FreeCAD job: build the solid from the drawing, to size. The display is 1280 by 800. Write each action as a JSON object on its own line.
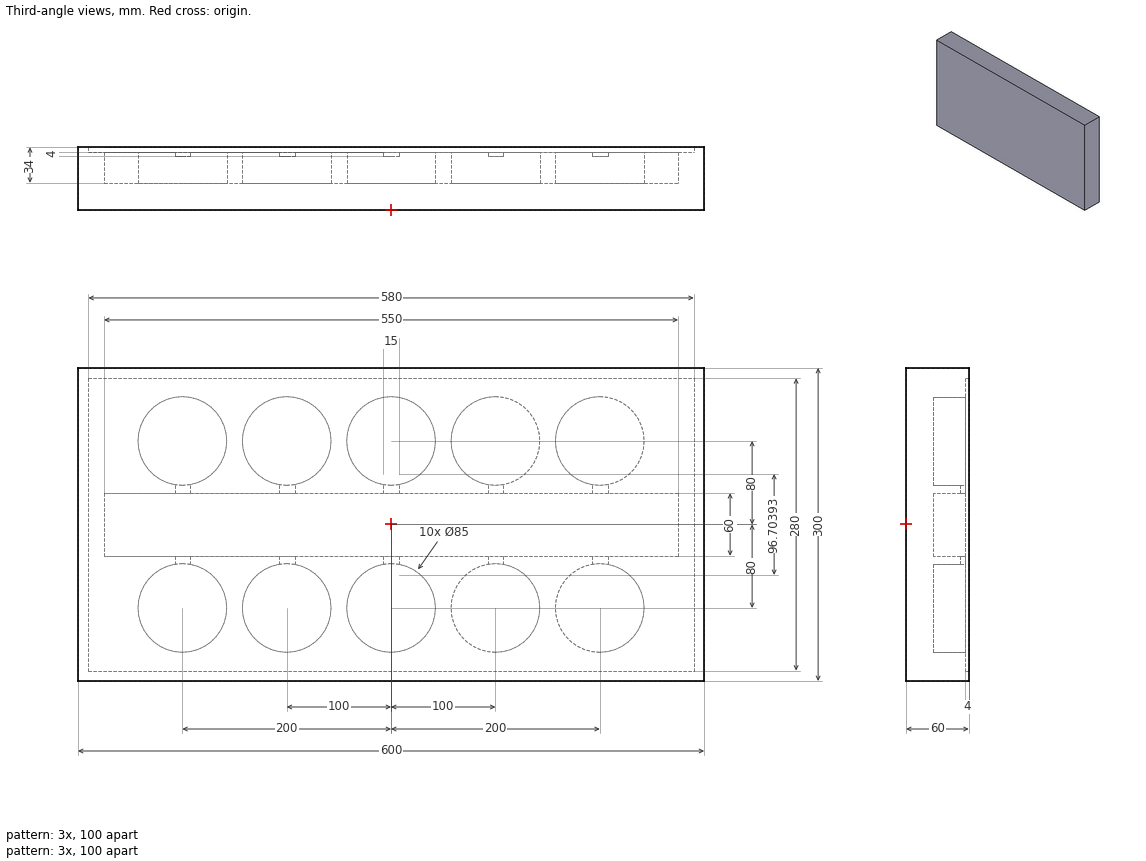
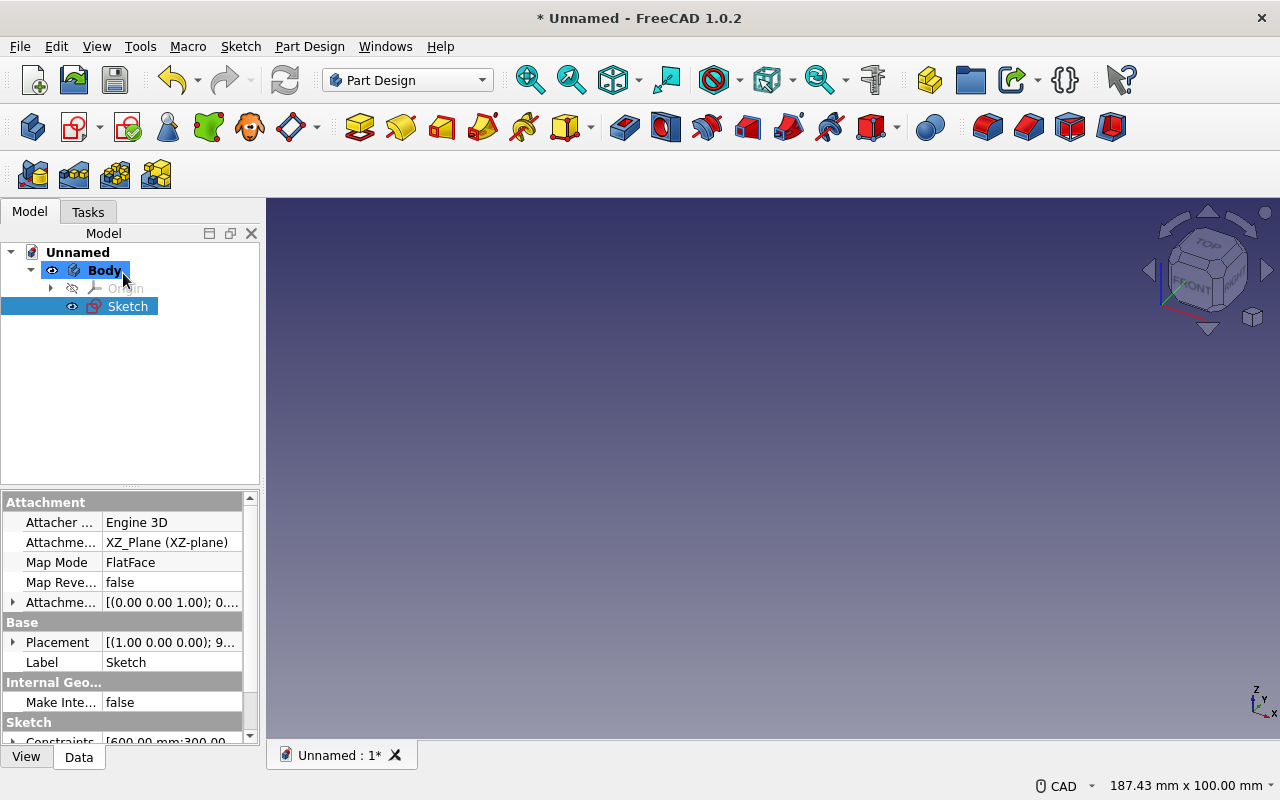
{"action": "left_click", "coordinate": [360, 128]}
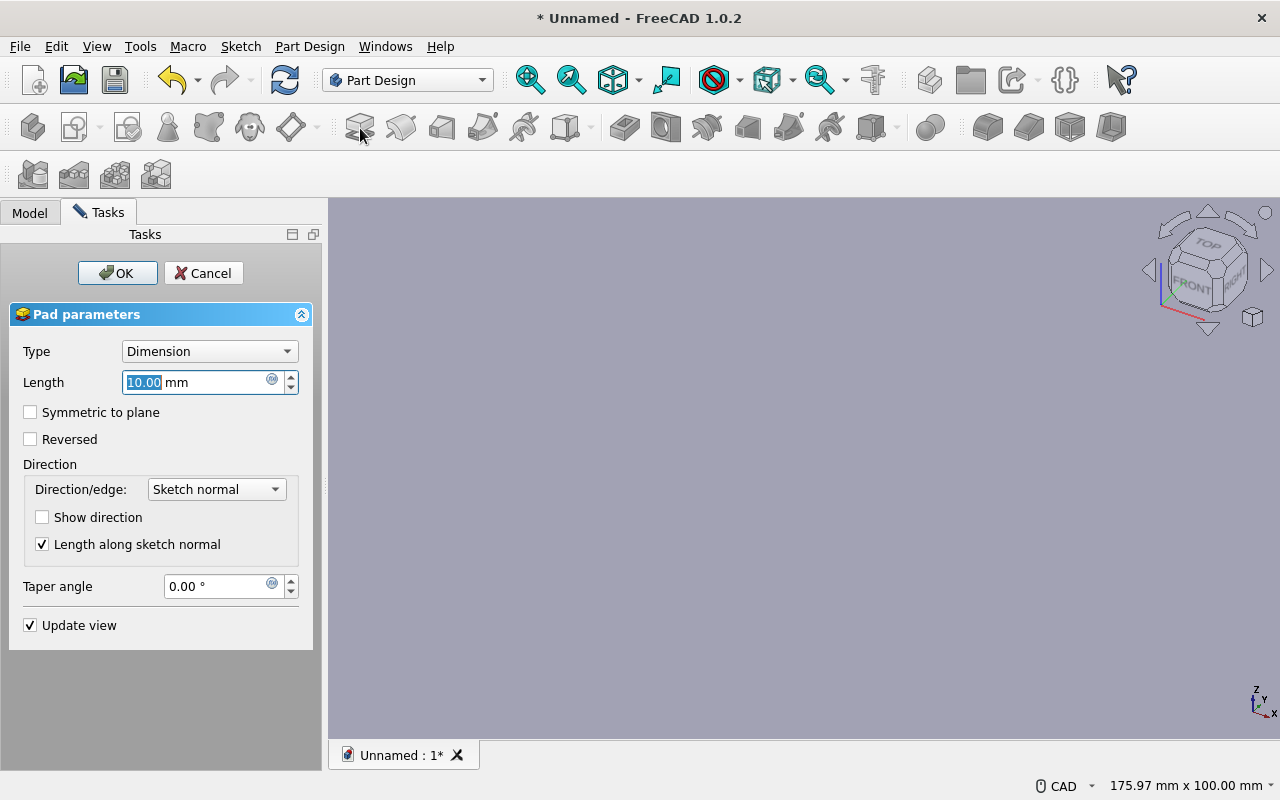
{"action": "type", "text": "60"}
{"action": "key", "text": "Tab"}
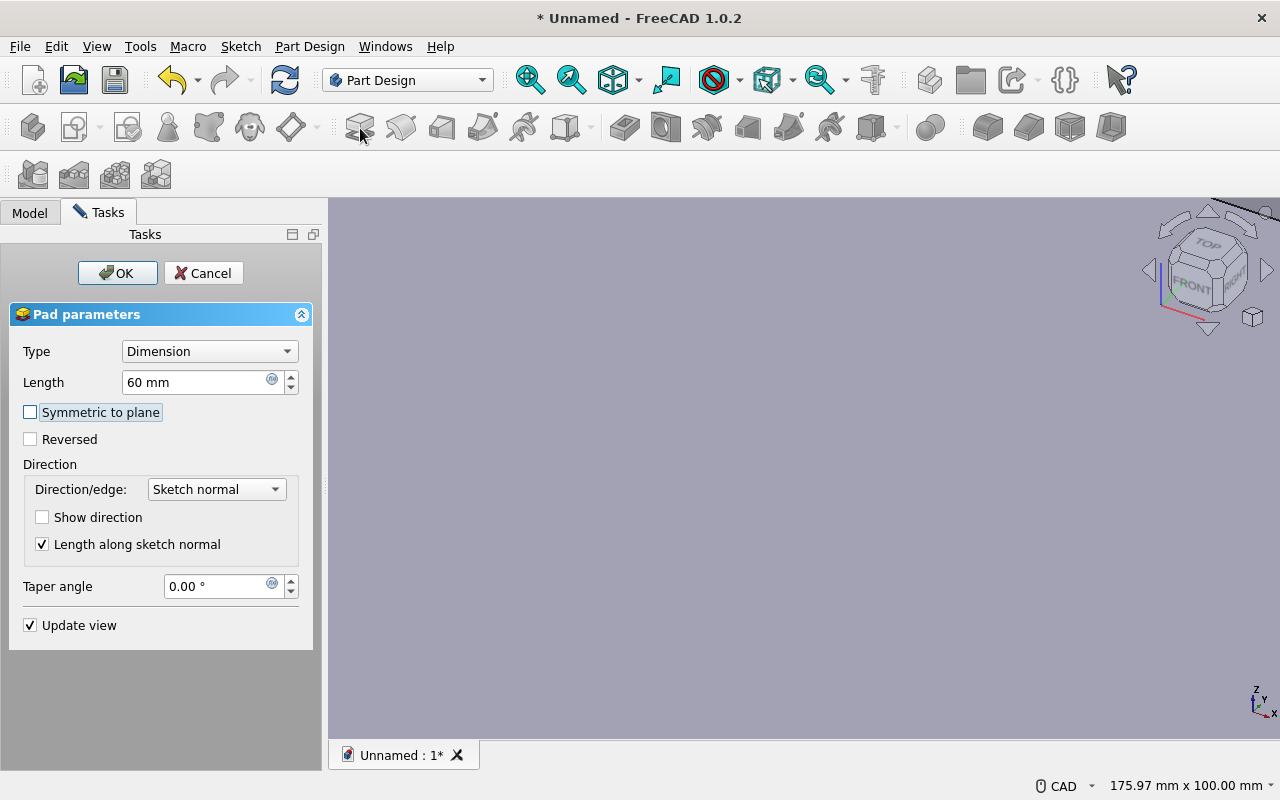
{"action": "left_click", "coordinate": [31, 439]}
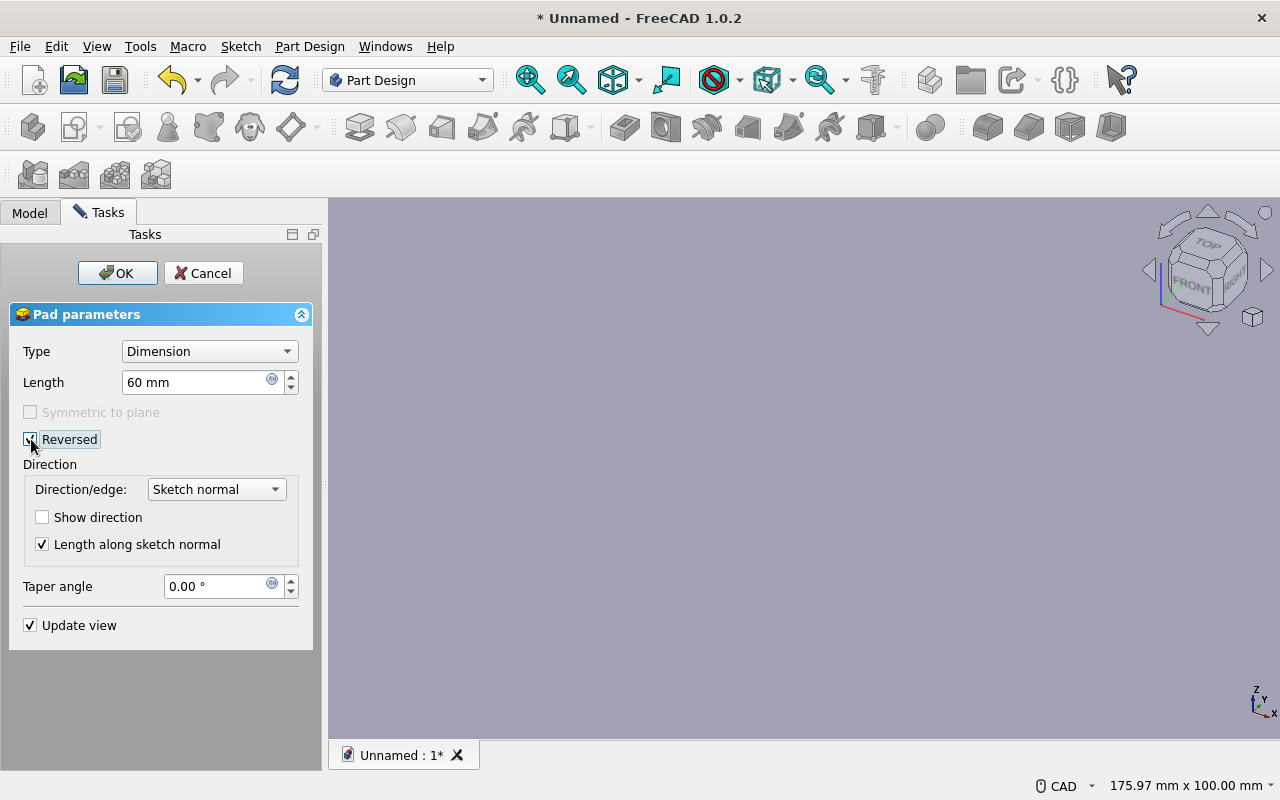
{"action": "left_click", "coordinate": [118, 273]}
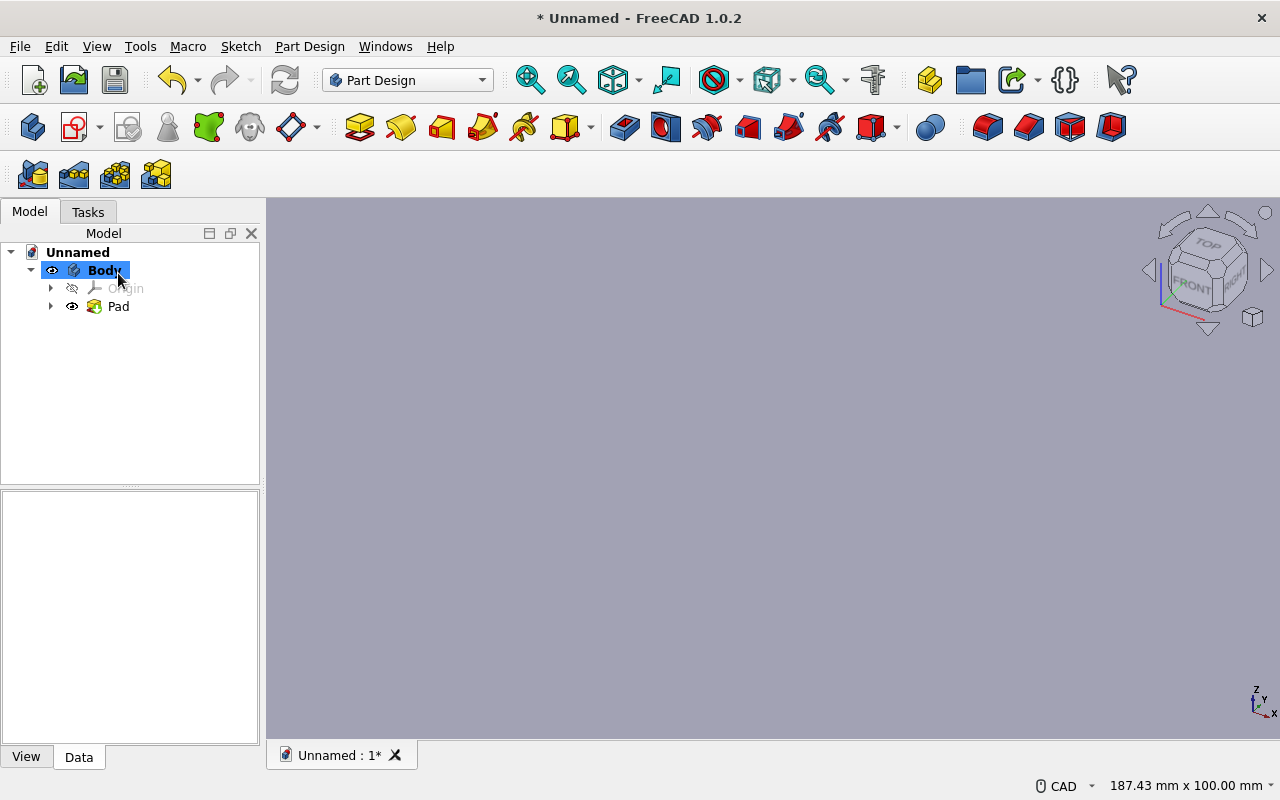
{"action": "left_click", "coordinate": [531, 80]}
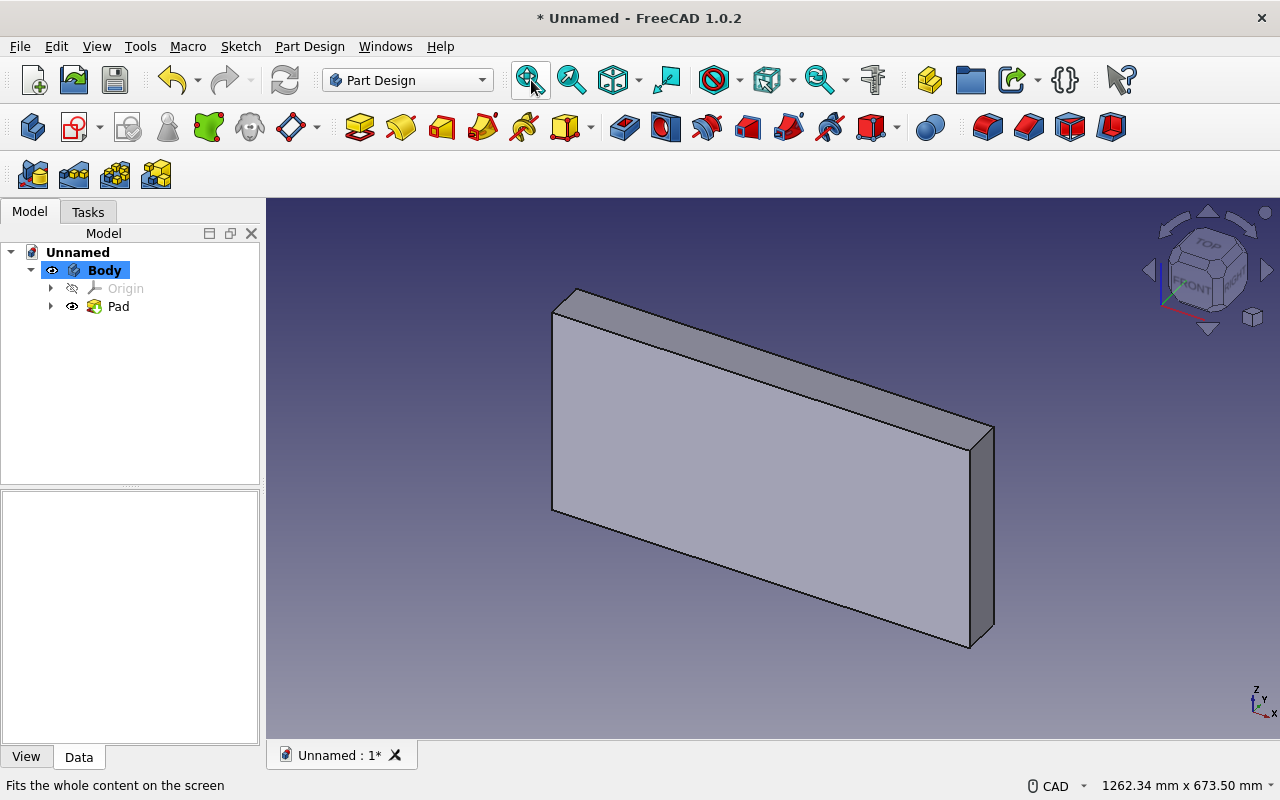
{"action": "key", "text": "4"}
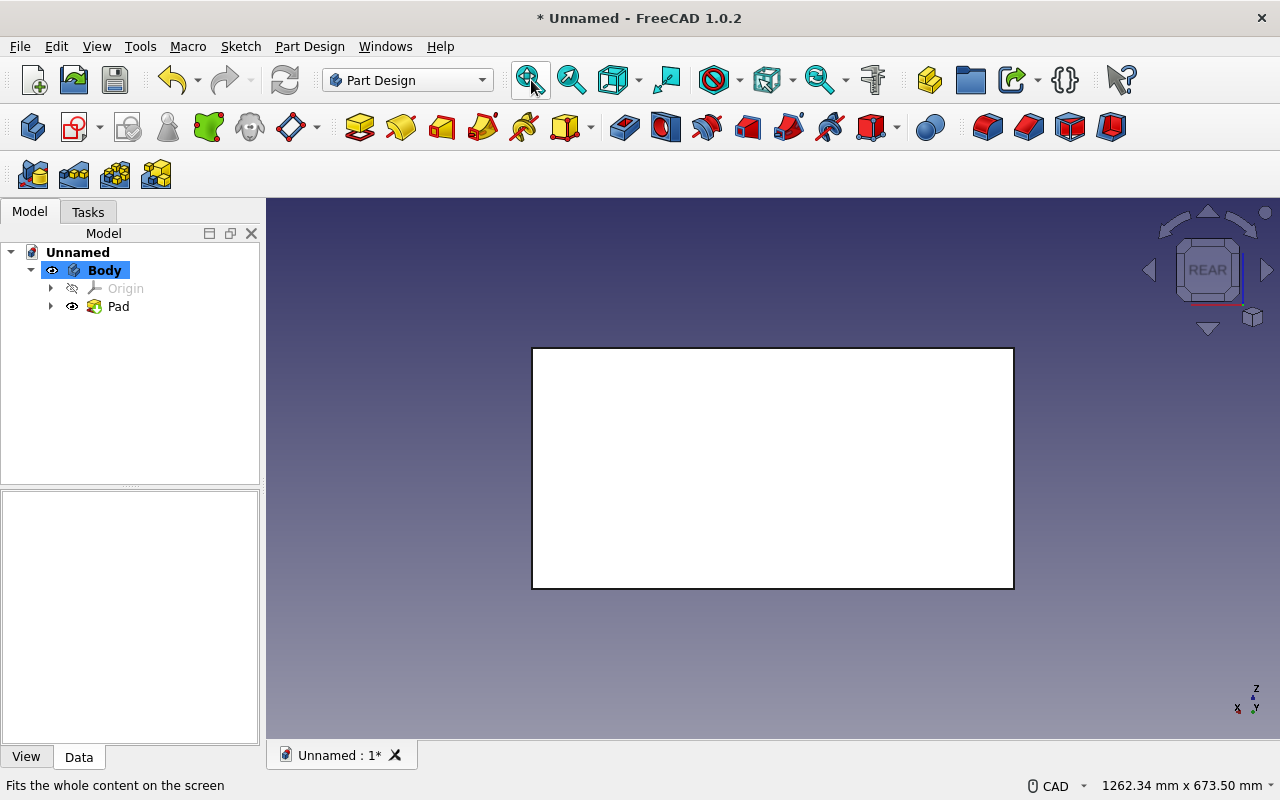
{"action": "left_click", "coordinate": [704, 468]}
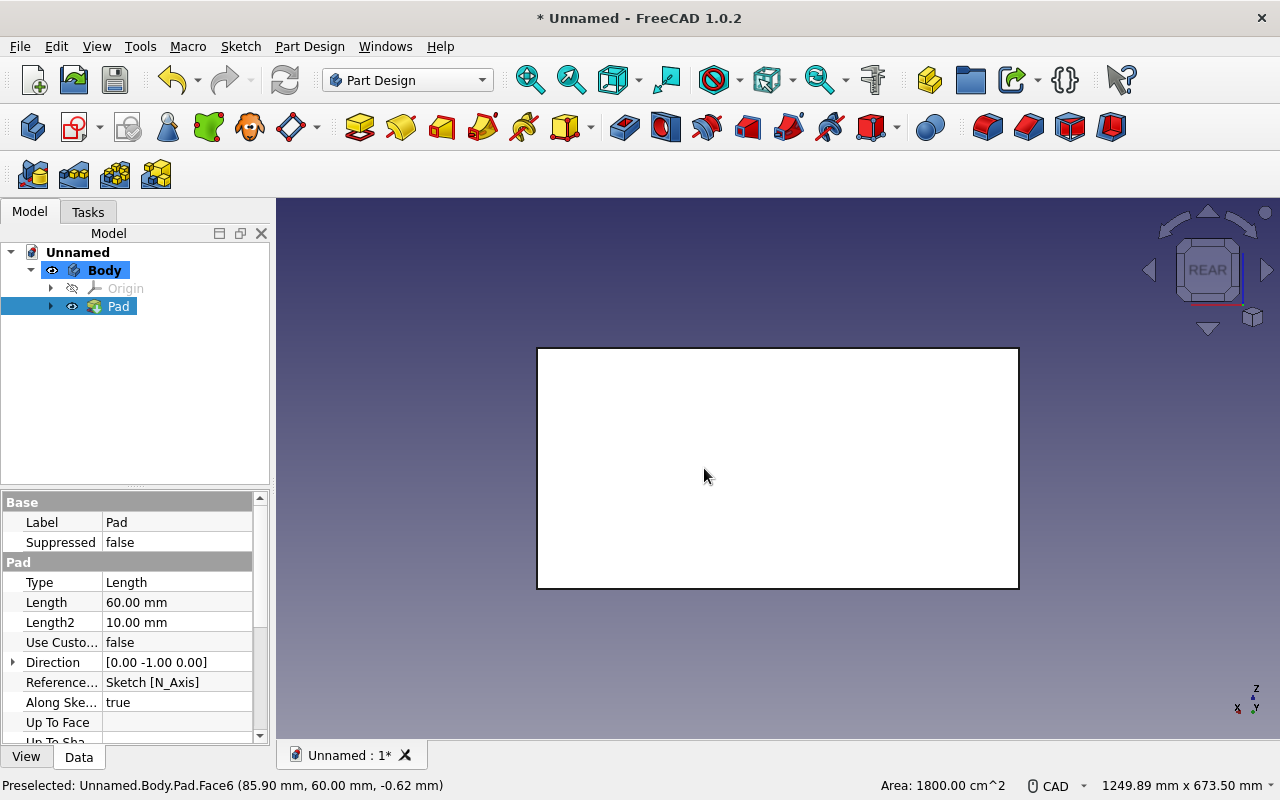
{"action": "left_click", "coordinate": [74, 128]}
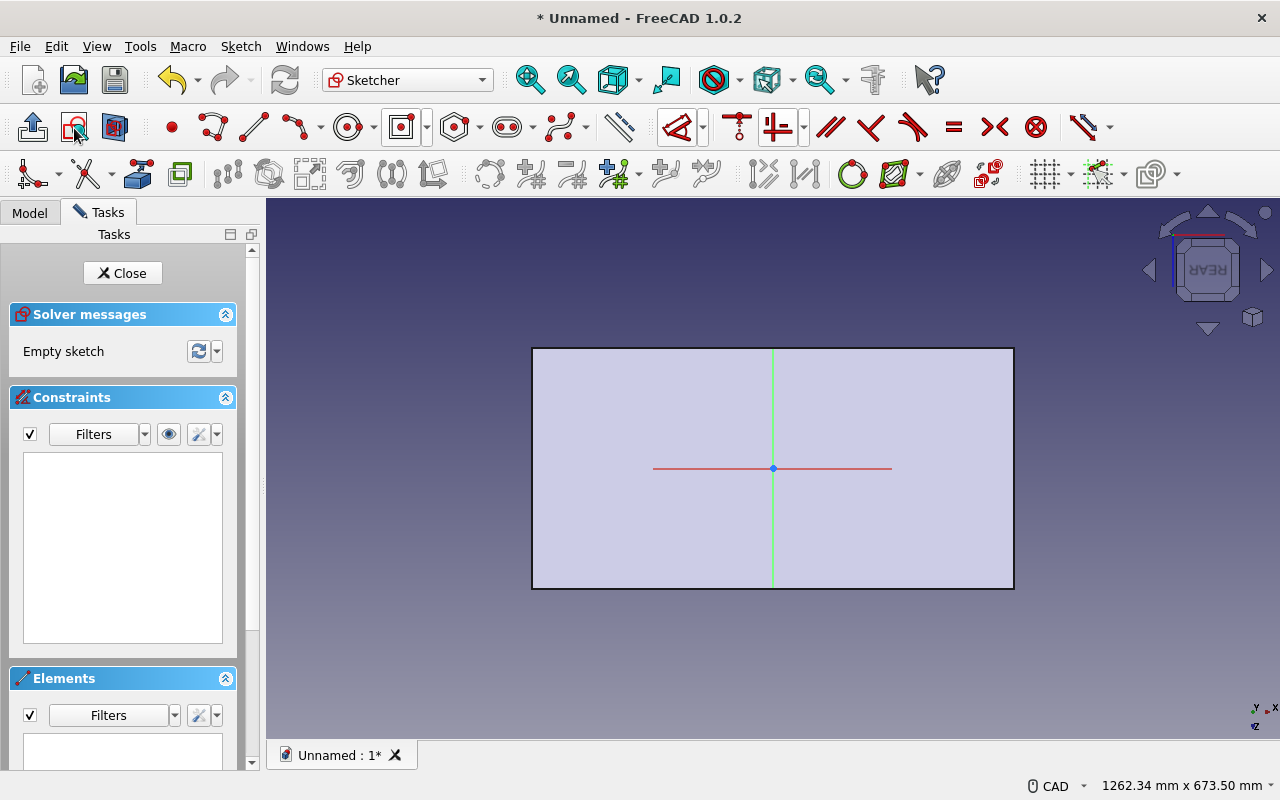
{"action": "left_click", "coordinate": [400, 128]}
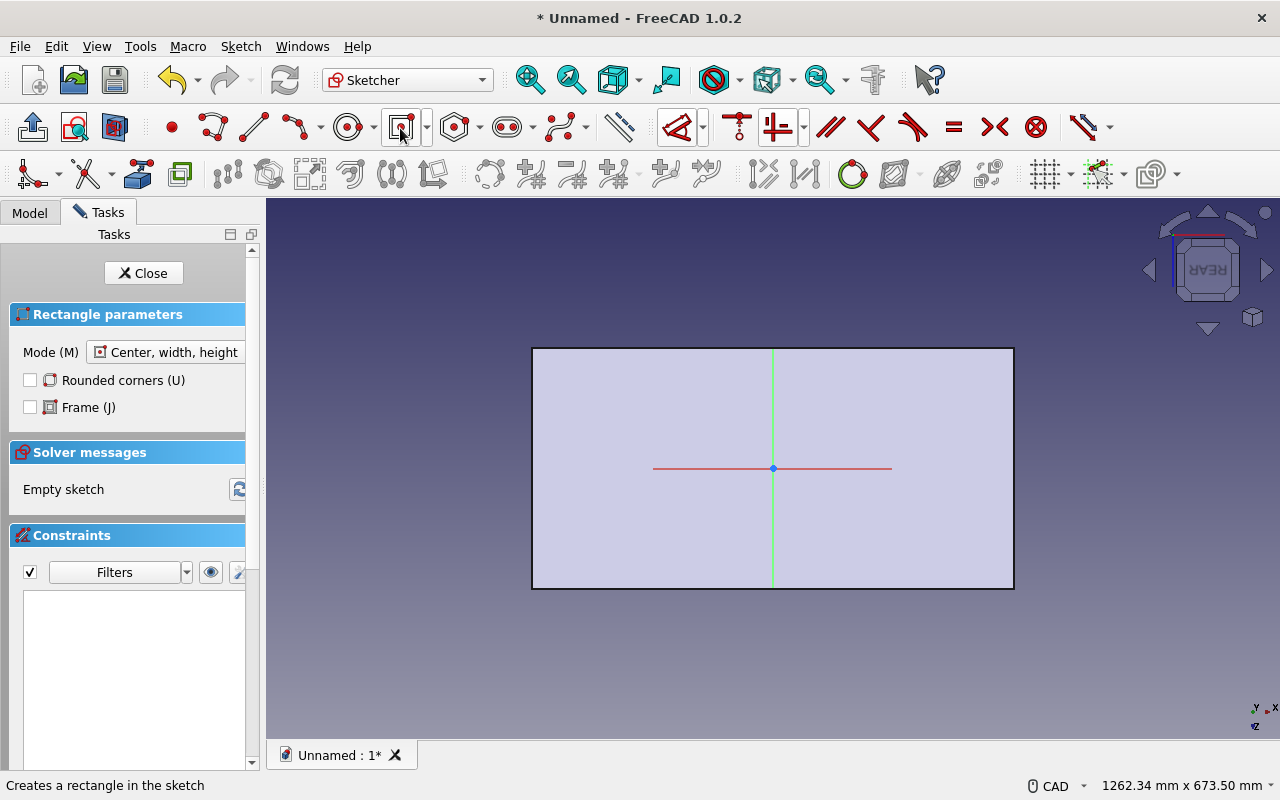
{"action": "left_click", "coordinate": [773, 468]}
{"action": "mouse_move", "coordinate": [994, 444]}